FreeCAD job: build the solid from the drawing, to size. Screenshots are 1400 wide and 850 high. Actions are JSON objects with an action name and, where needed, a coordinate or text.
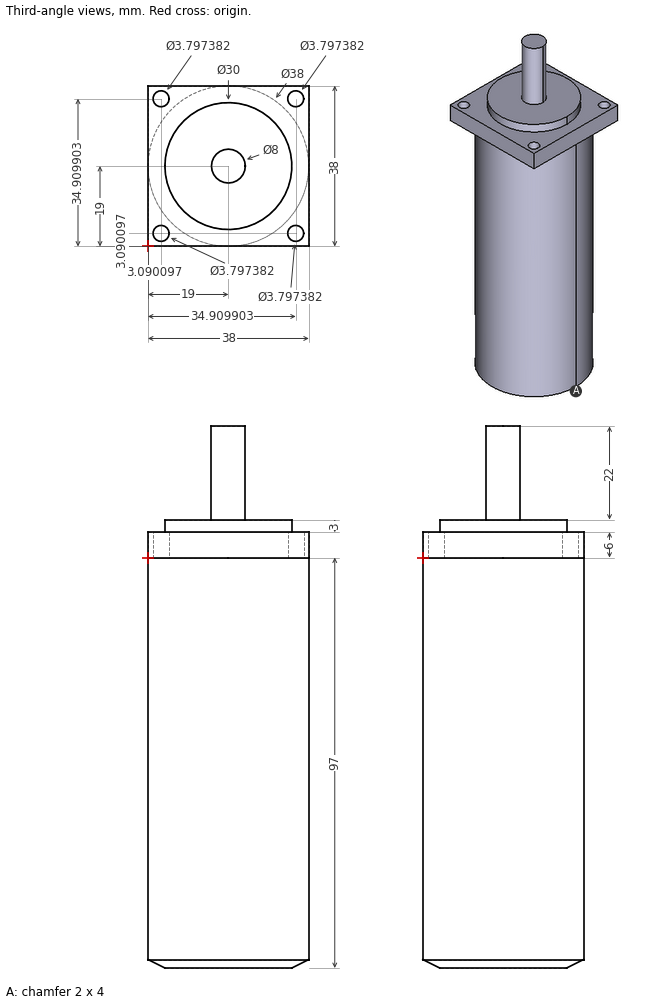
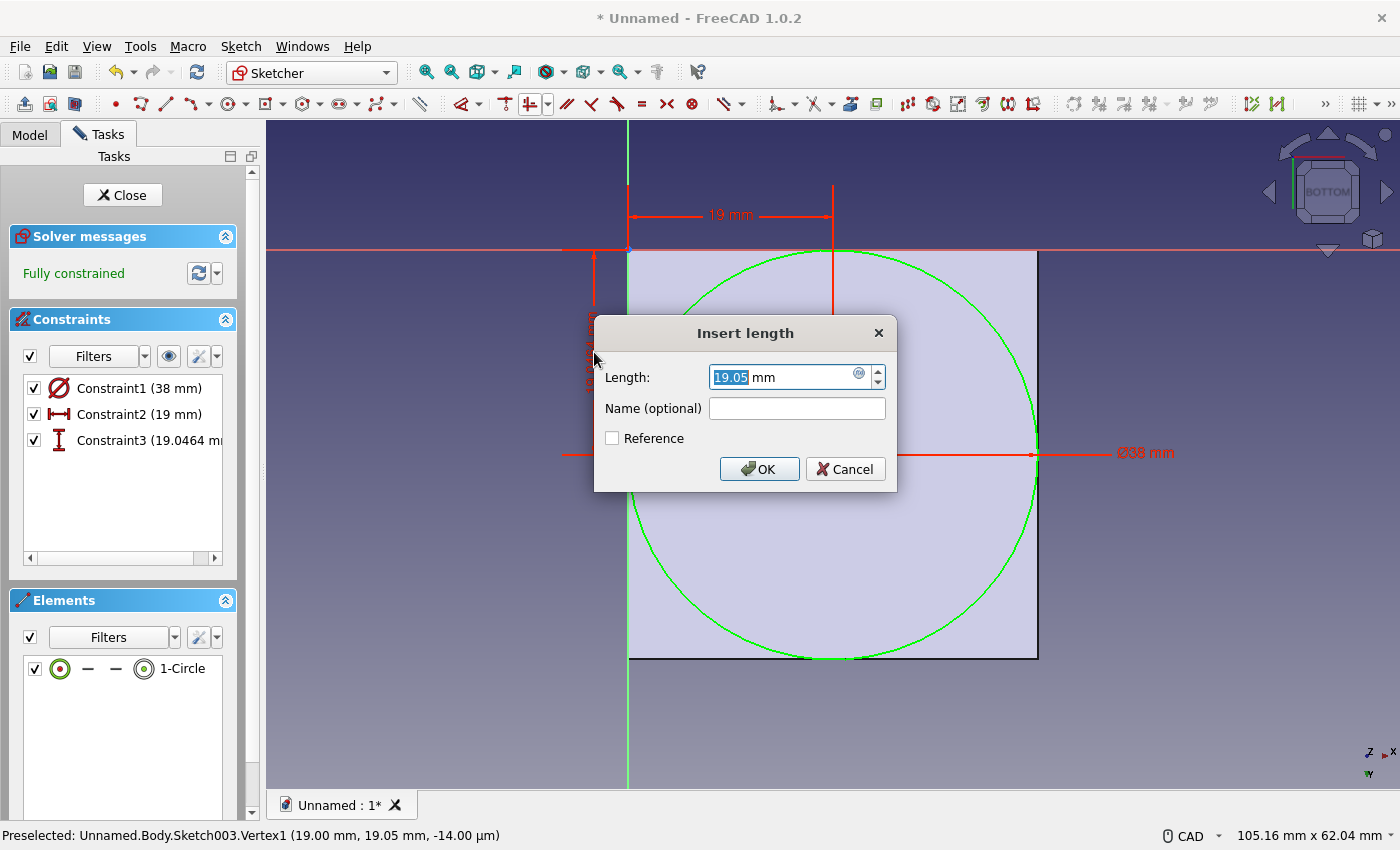
{"action": "type", "text": "19"}
{"action": "key", "text": "Return"}
{"action": "key", "text": "Escape"}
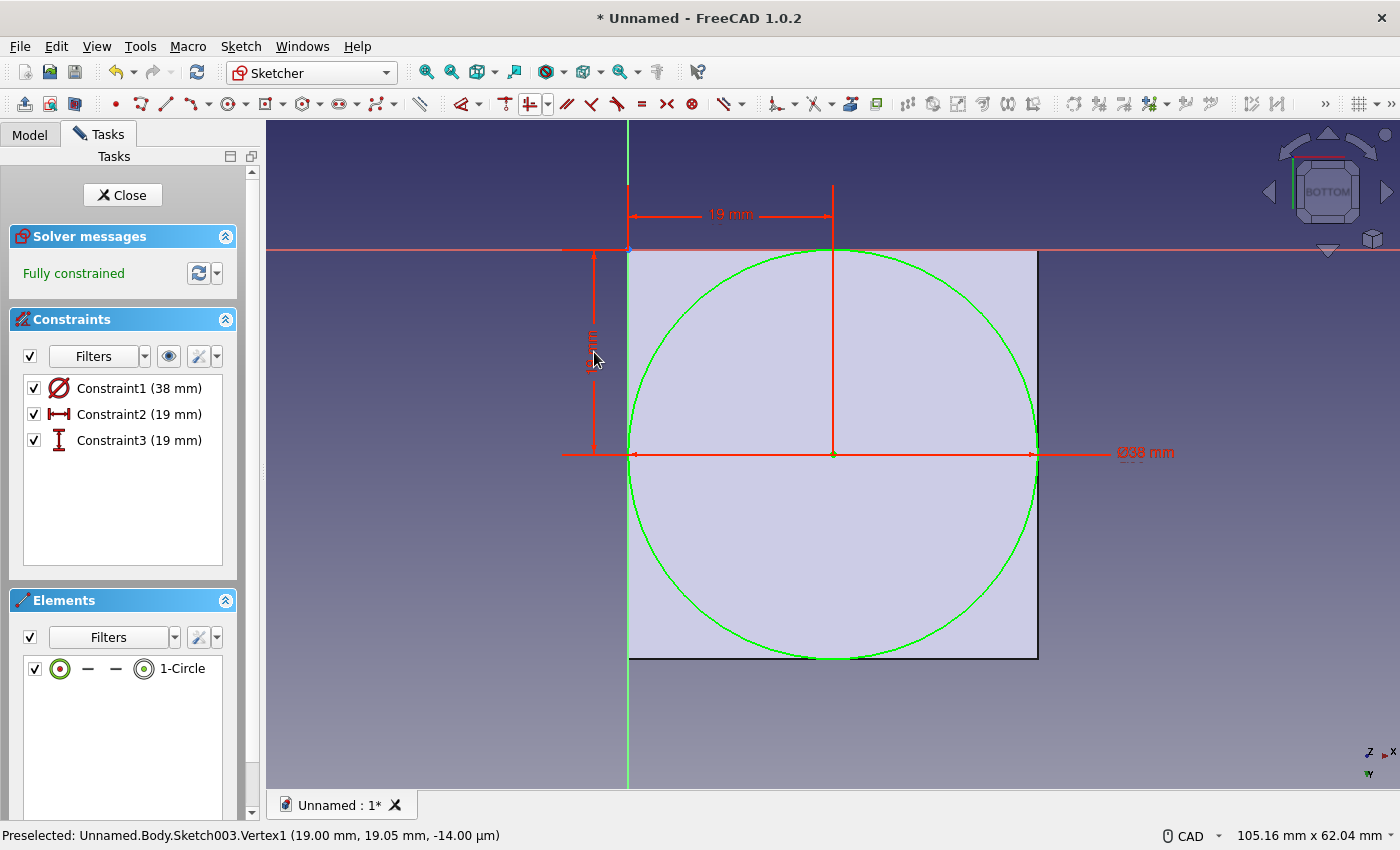
{"action": "left_click", "coordinate": [123, 195]}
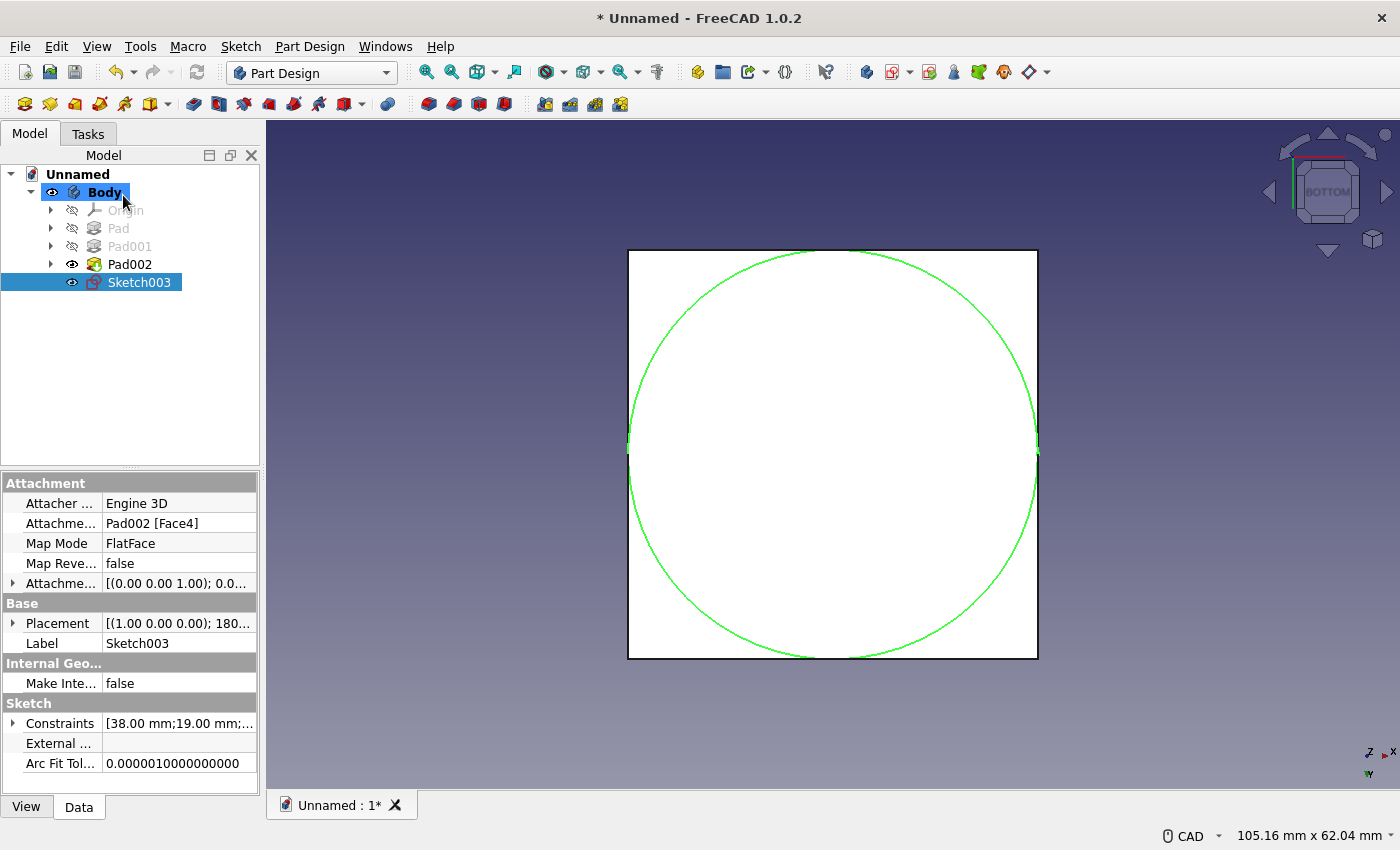
{"action": "left_click", "coordinate": [25, 104]}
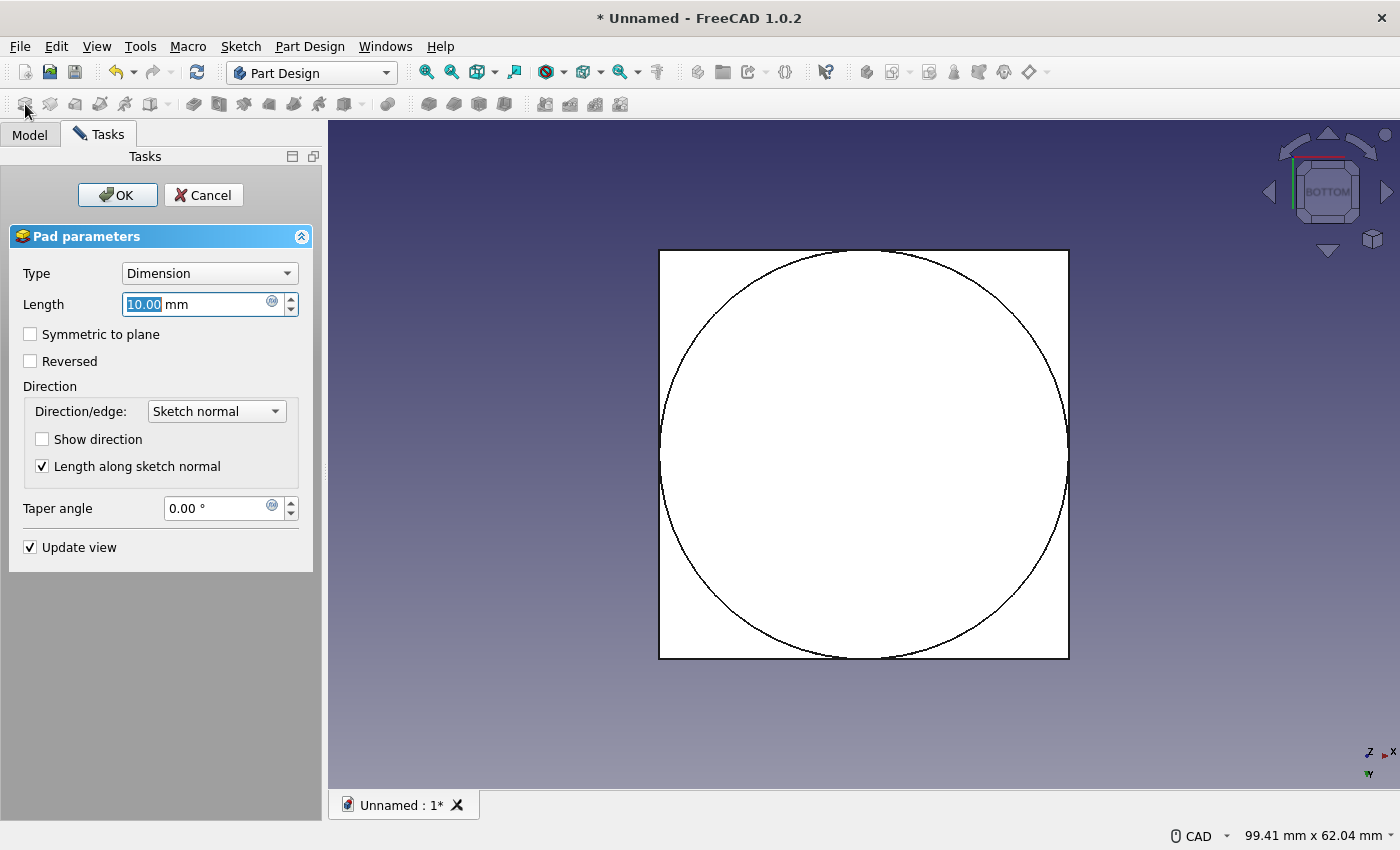
{"action": "type", "text": "97"}
{"action": "key", "text": "Tab"}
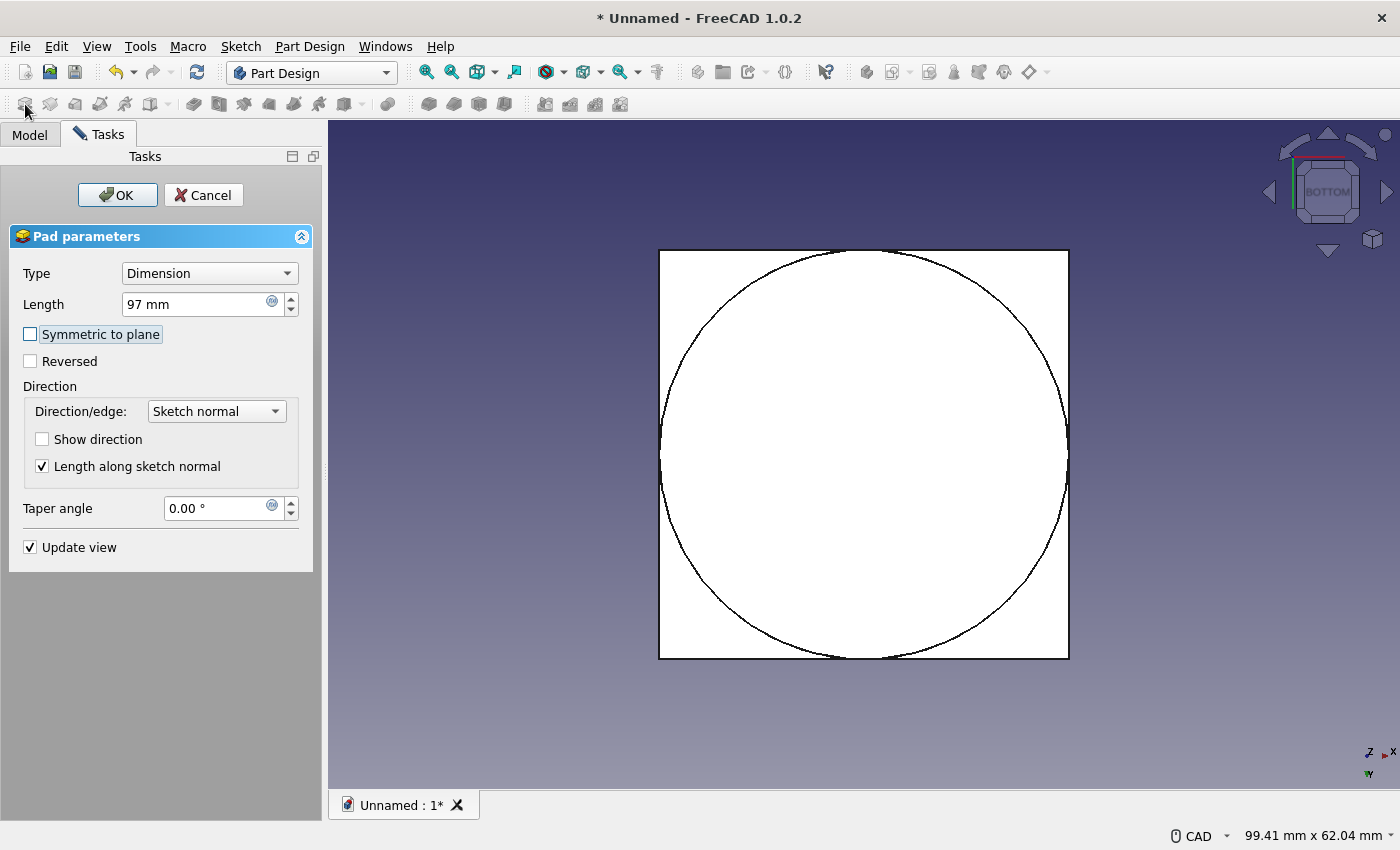
{"action": "left_click", "coordinate": [118, 195]}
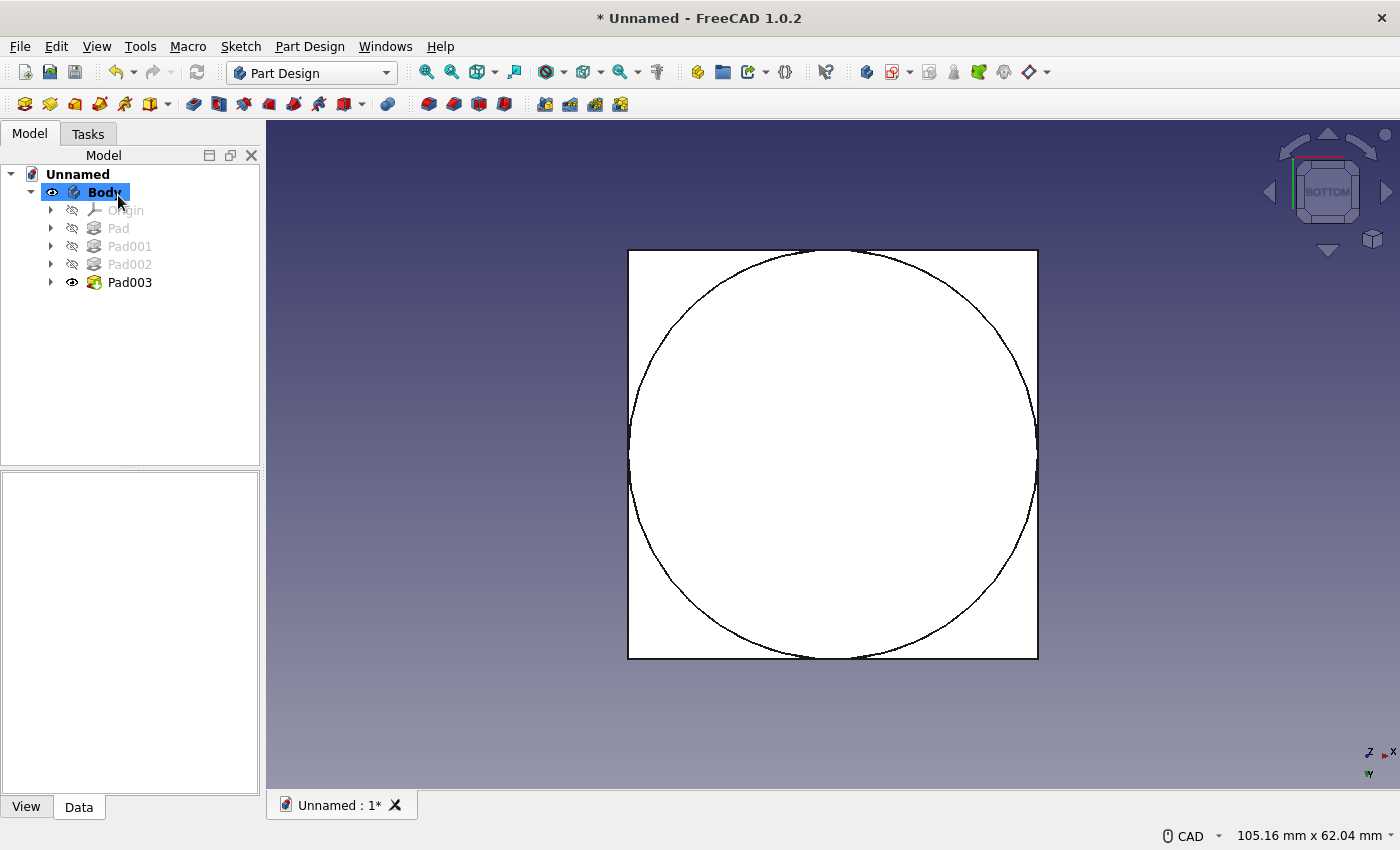
{"action": "key", "text": "0"}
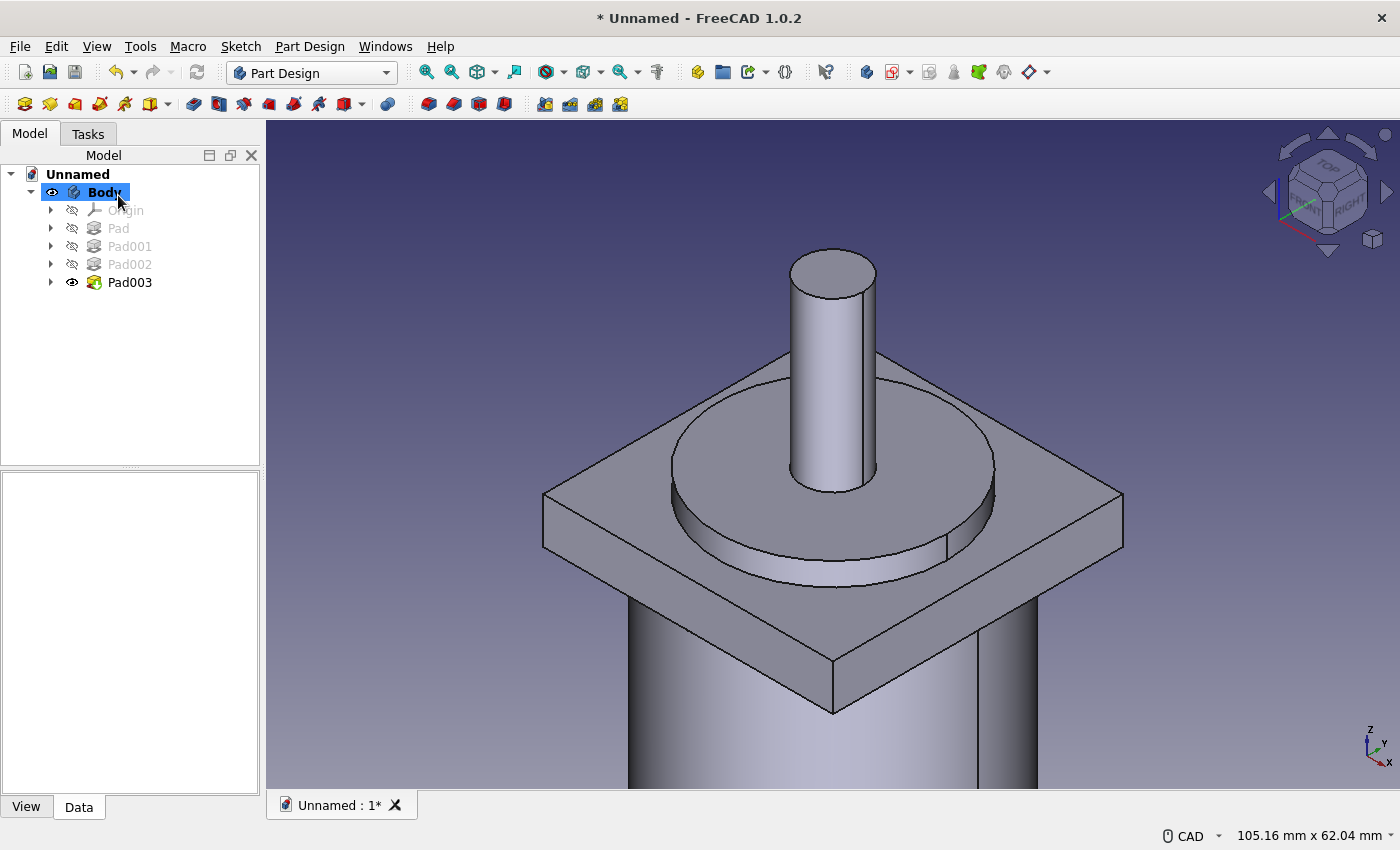
{"action": "key", "text": "v f"}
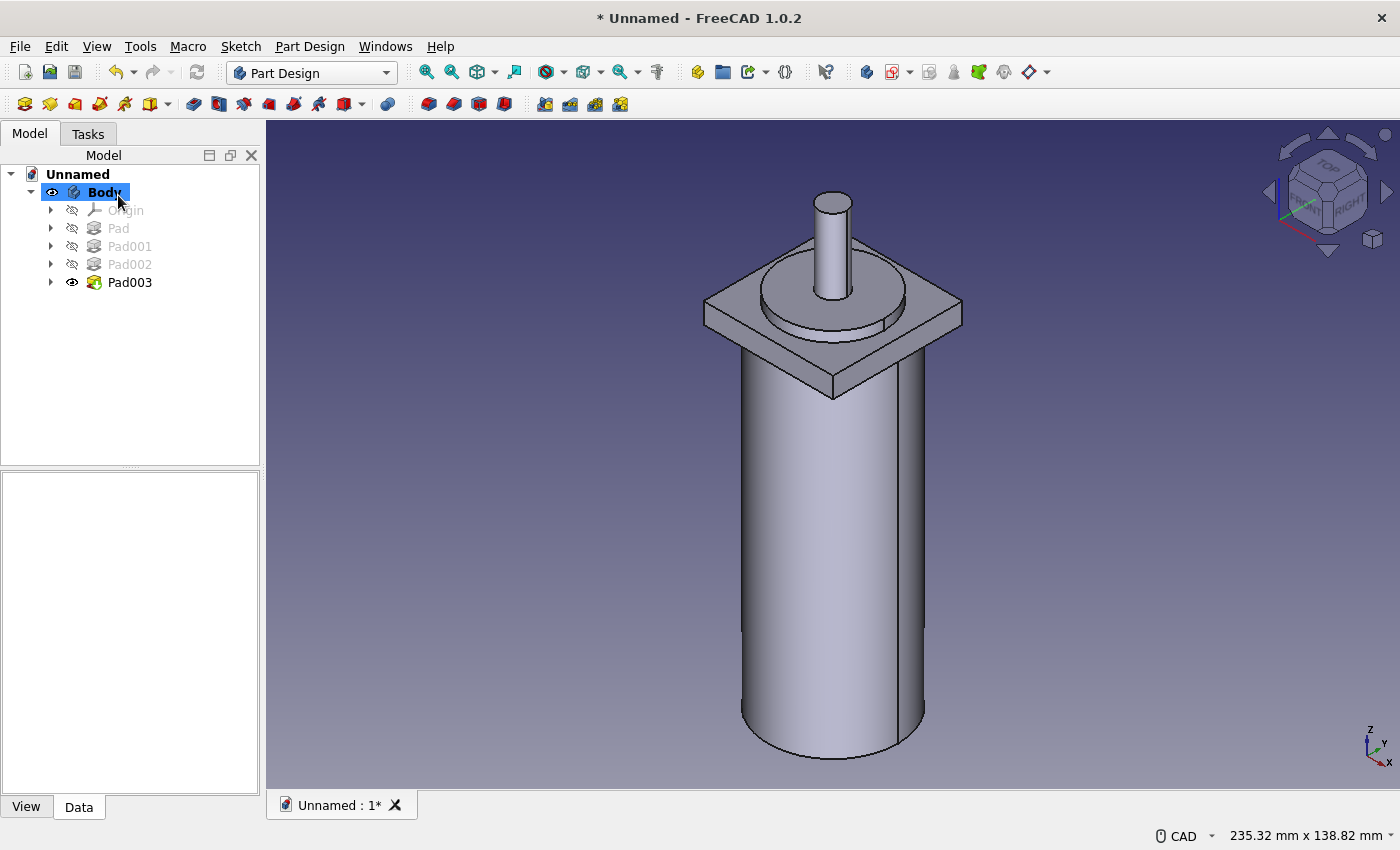
{"action": "left_click", "coordinate": [944, 300]}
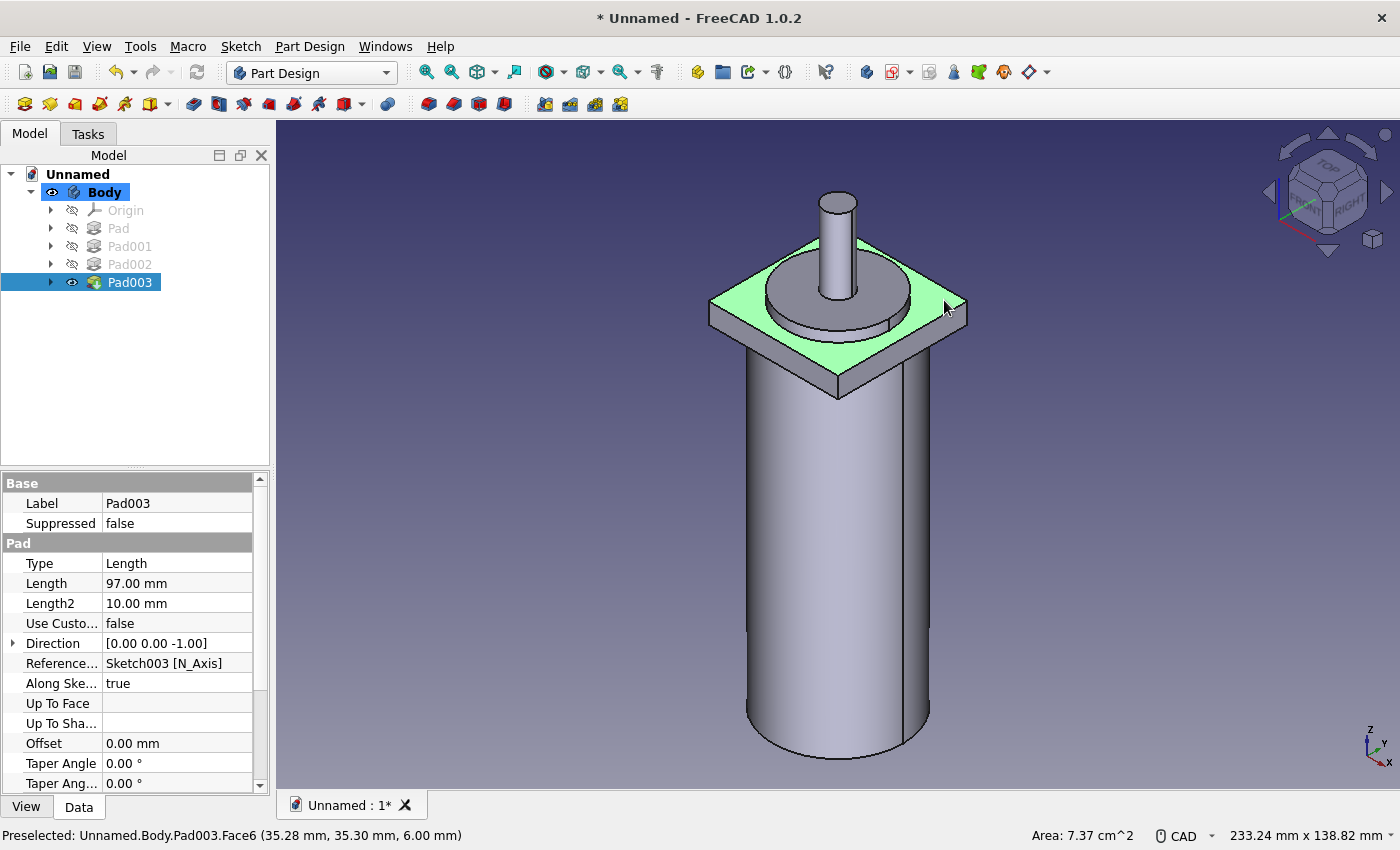
{"action": "left_click", "coordinate": [892, 72]}